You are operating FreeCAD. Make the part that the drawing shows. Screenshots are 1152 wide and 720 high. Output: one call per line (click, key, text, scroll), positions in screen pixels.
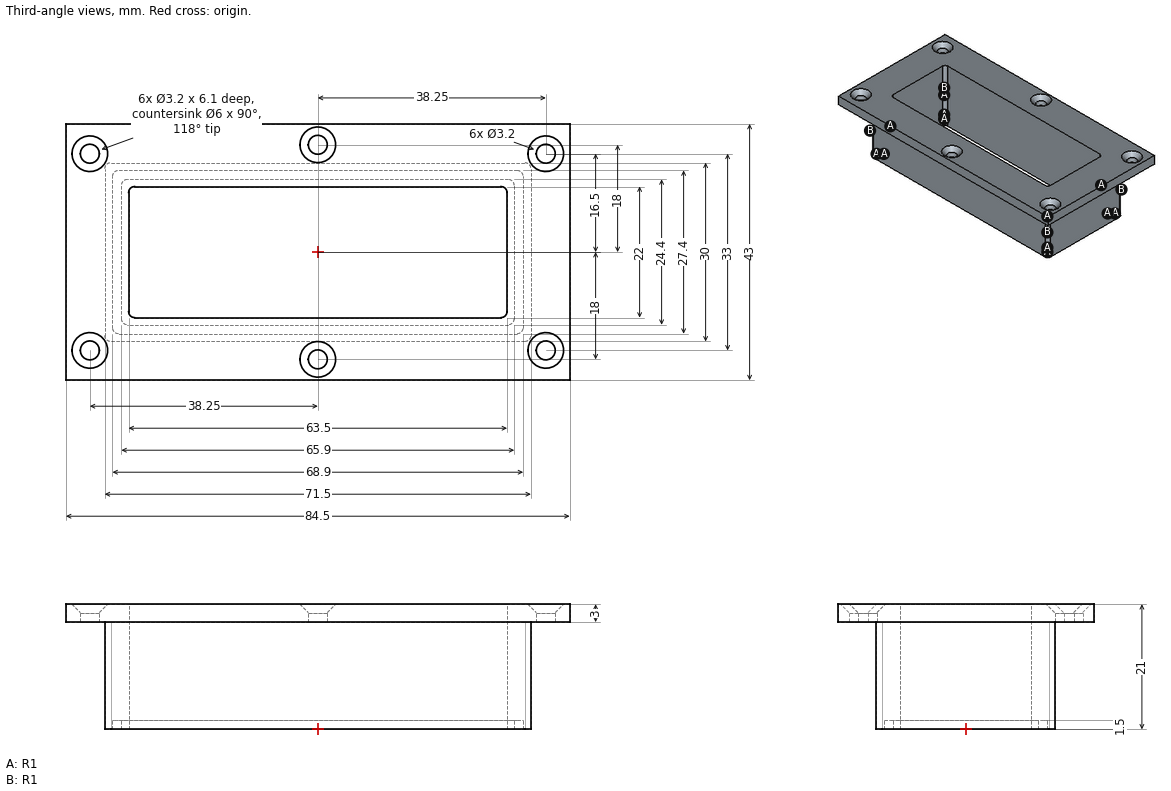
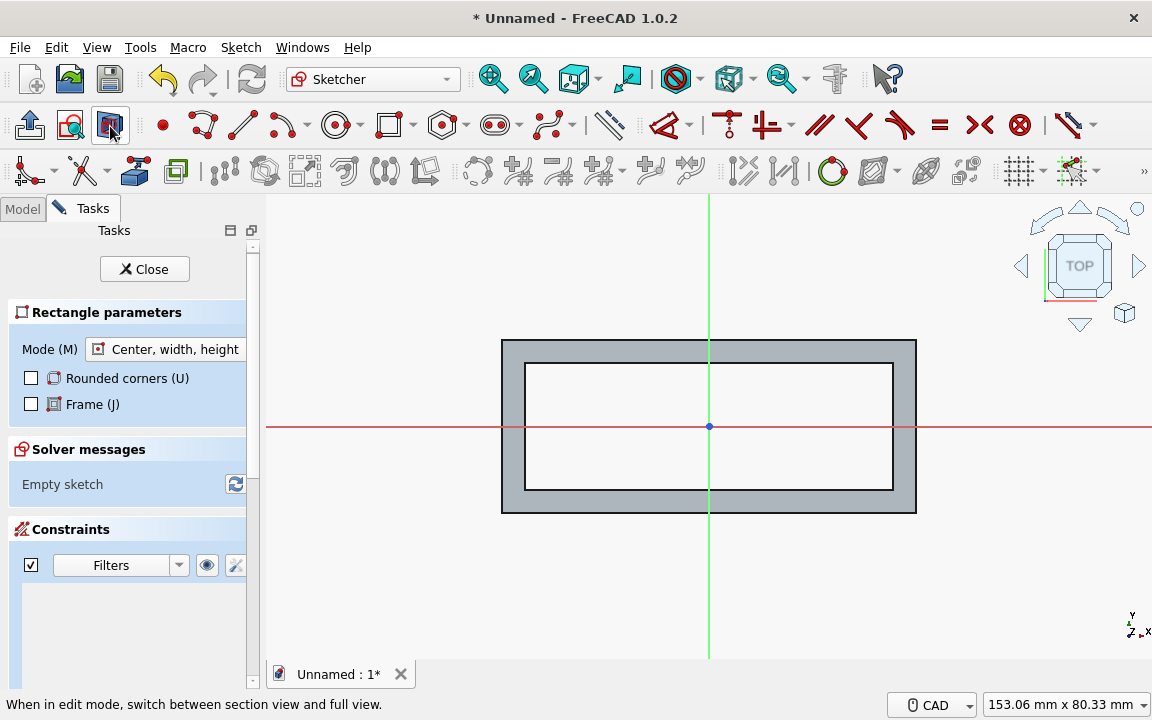
click(709, 426)
click(908, 347)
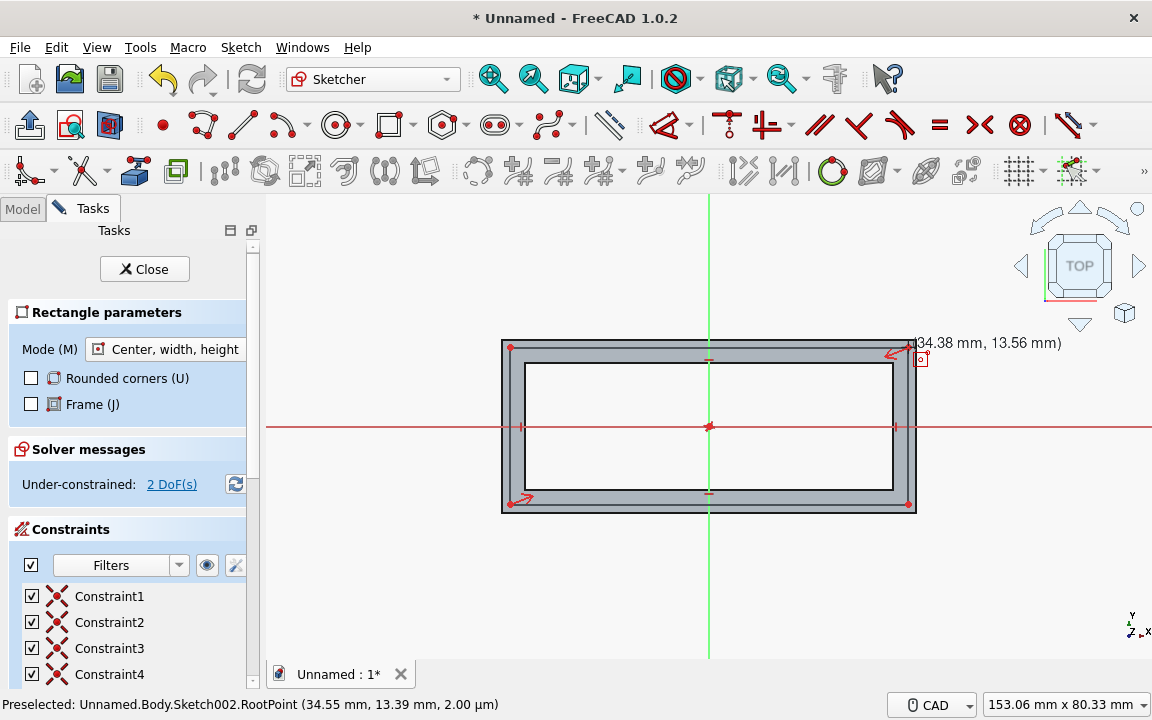
click(709, 426)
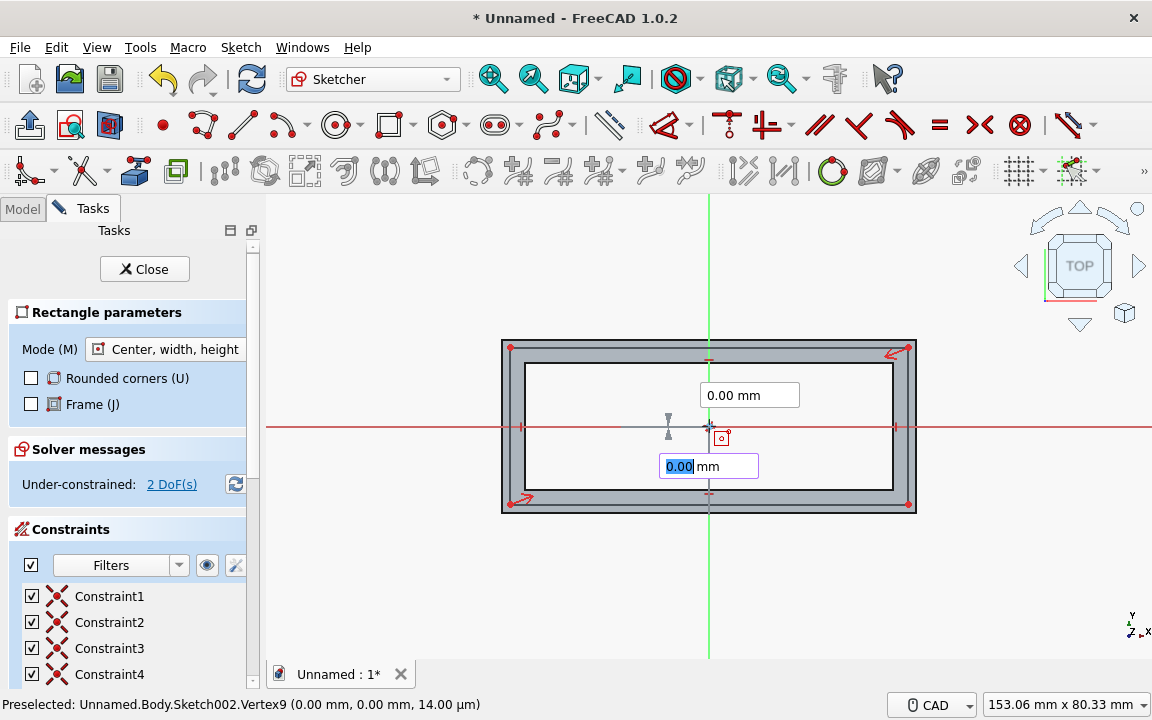
scroll(900, 356, up, 4)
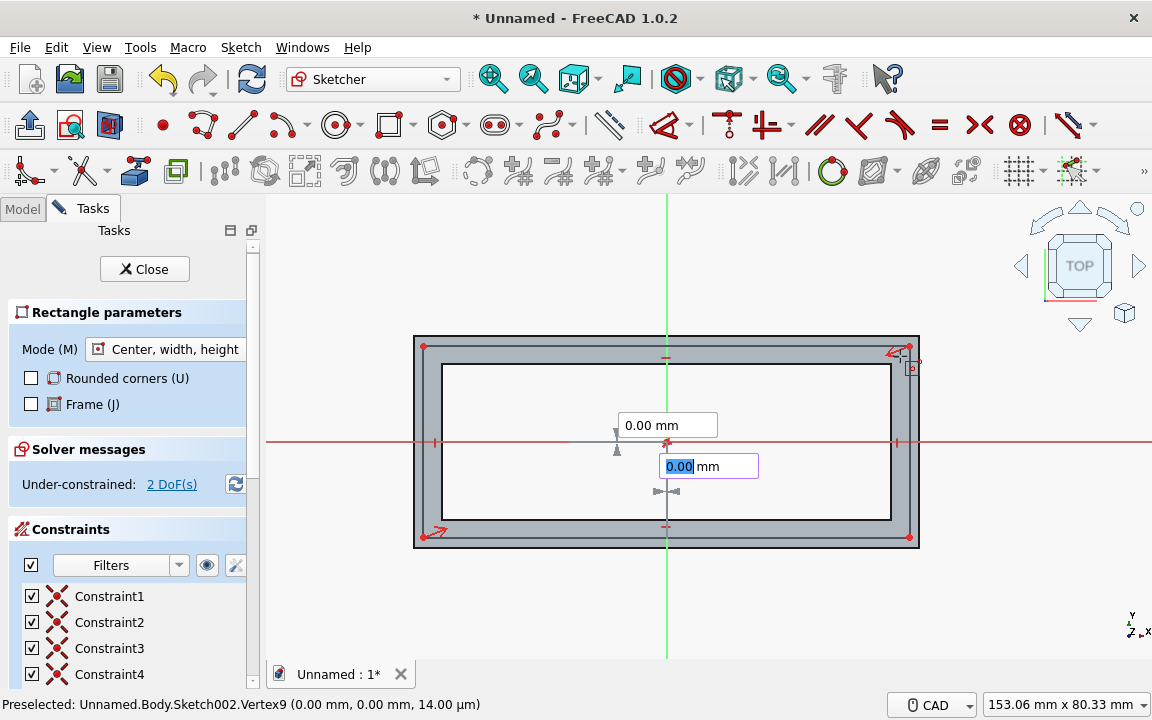
click(899, 355)
key(Escape)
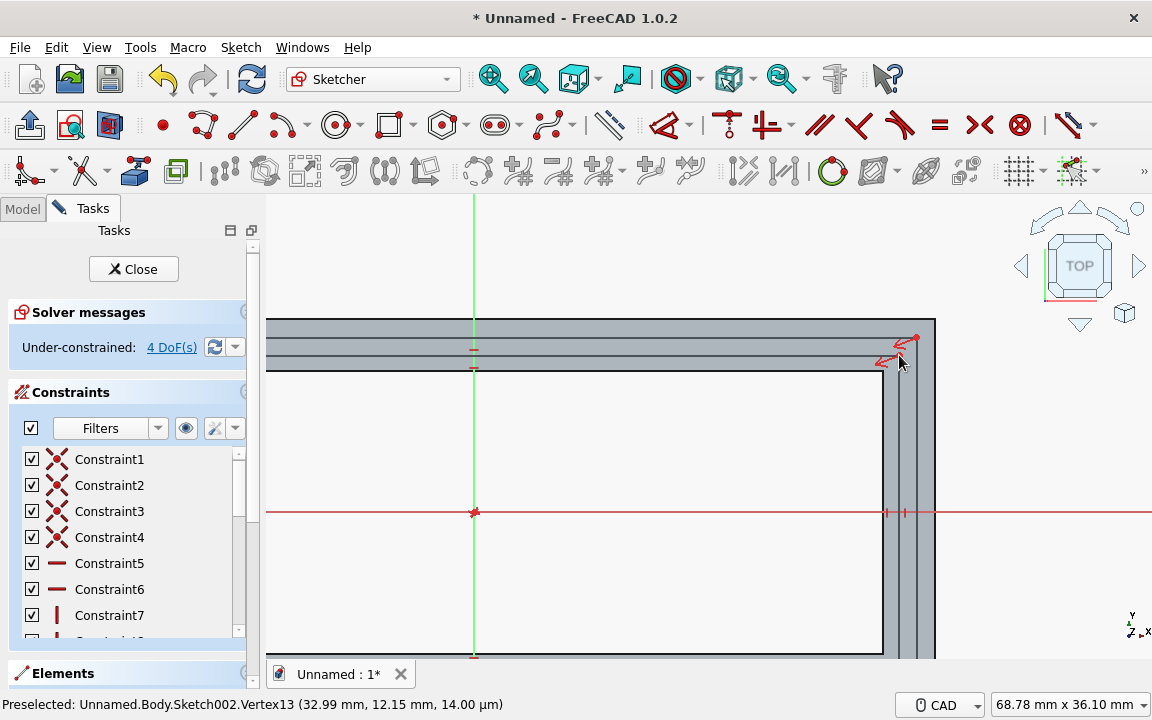
click(664, 126)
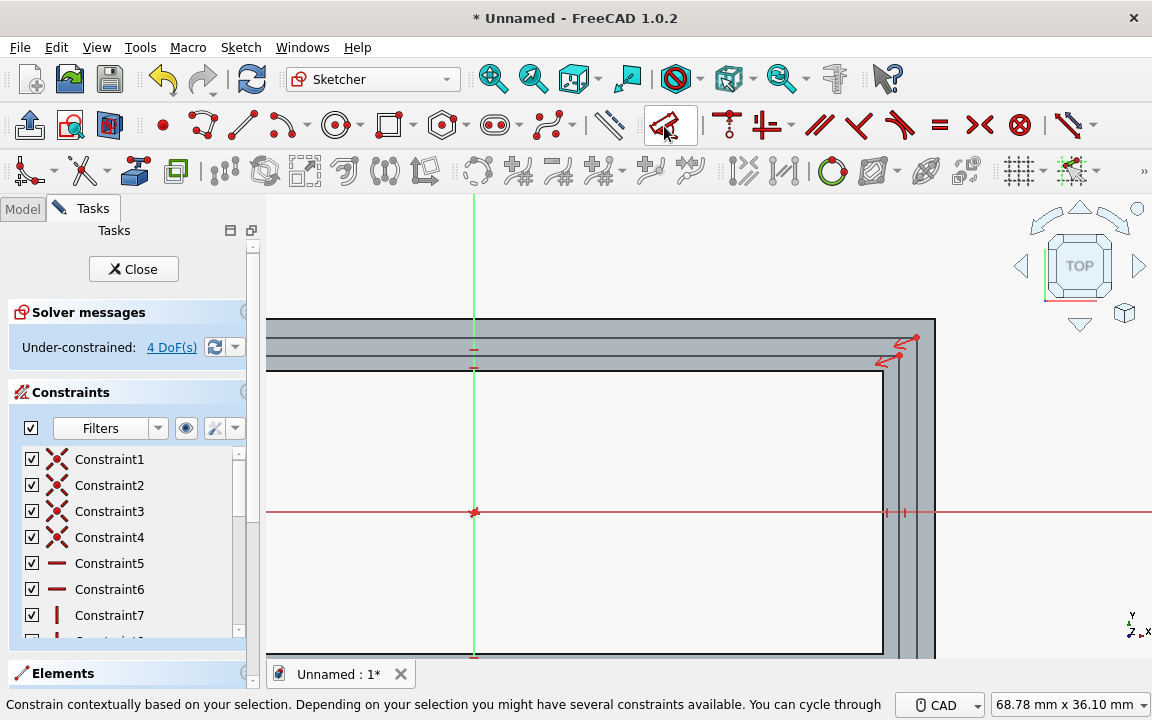
scroll(843, 322, down, 3)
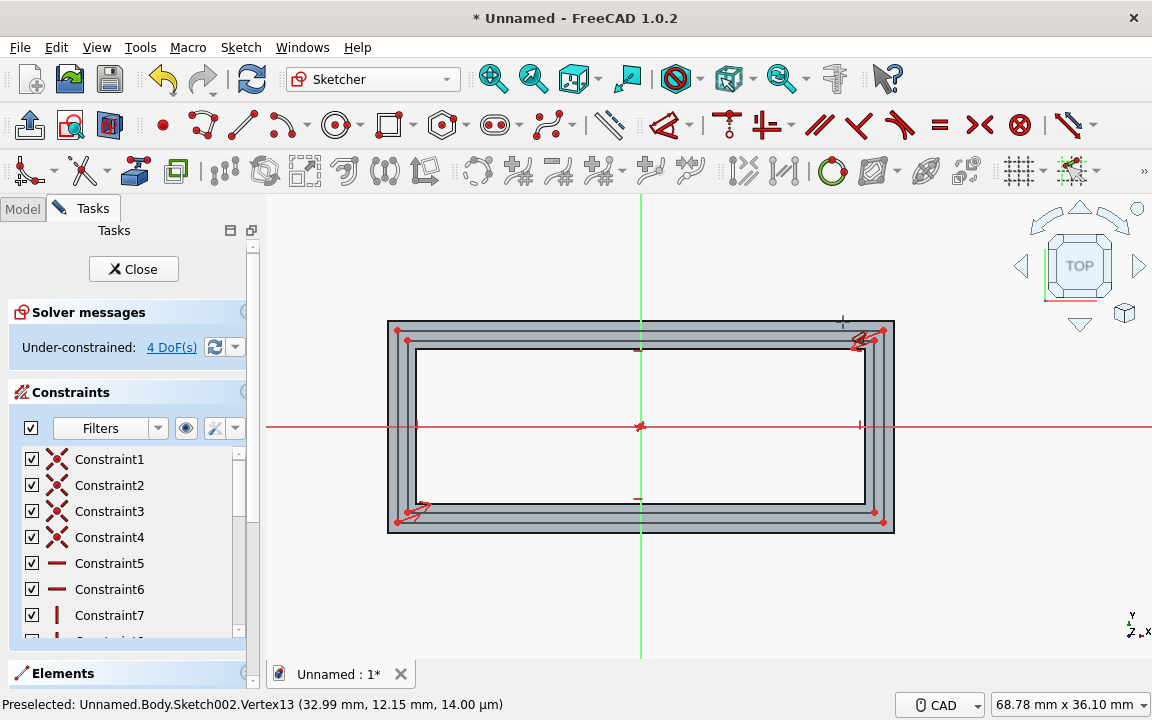
scroll(544, 523, up, 2)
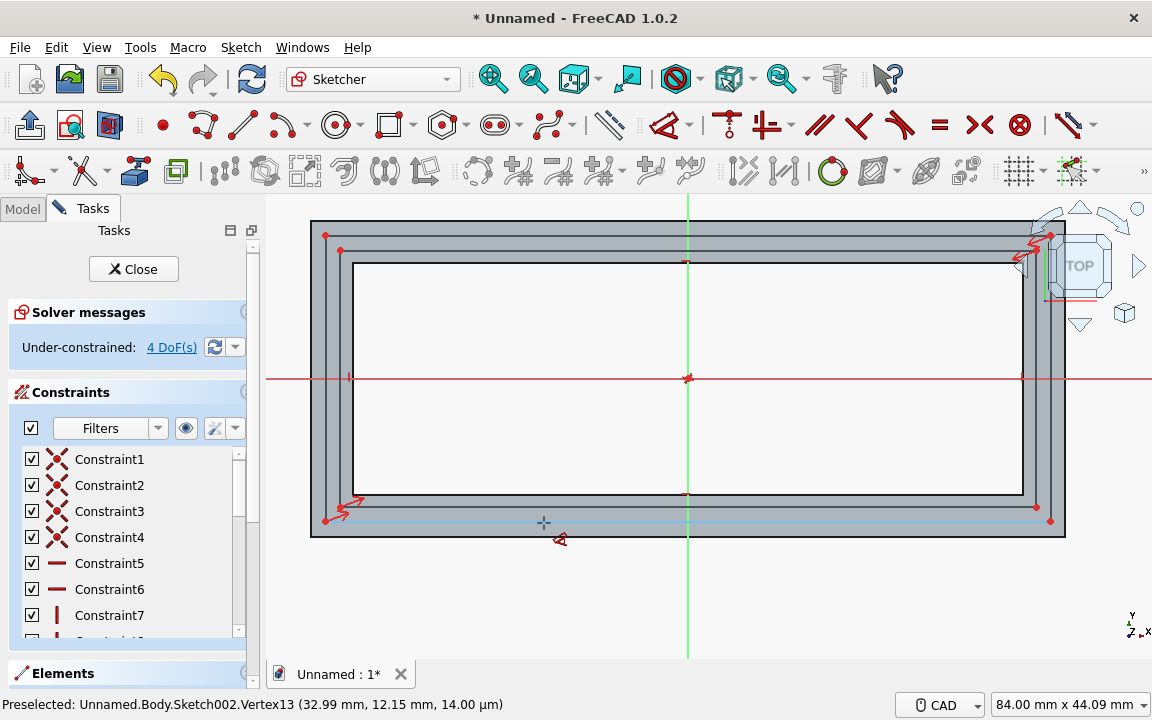
click(543, 522)
click(656, 556)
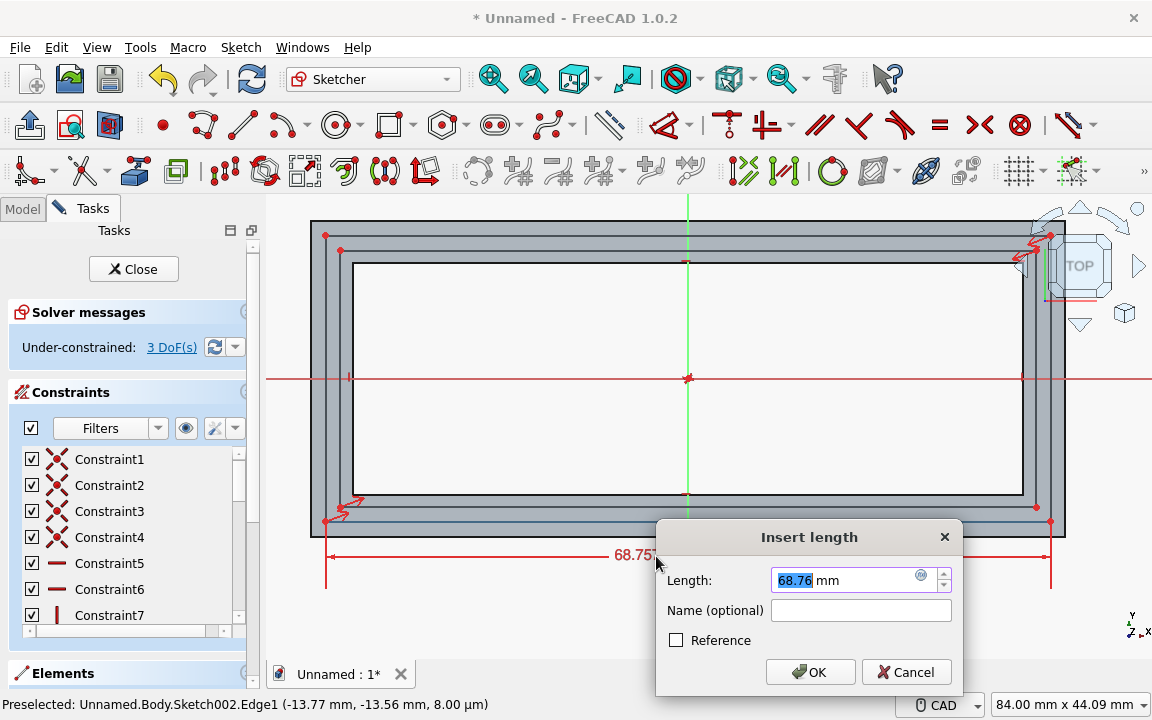
text(68.9)
key(Return)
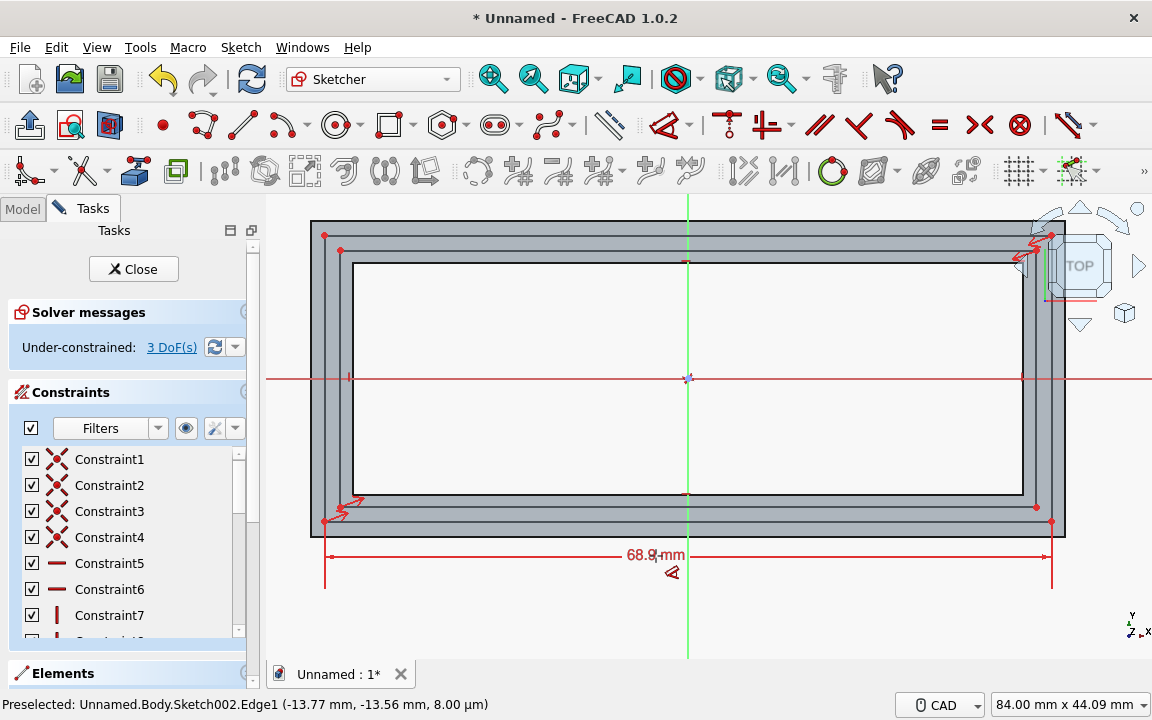
scroll(543, 523, down, 2)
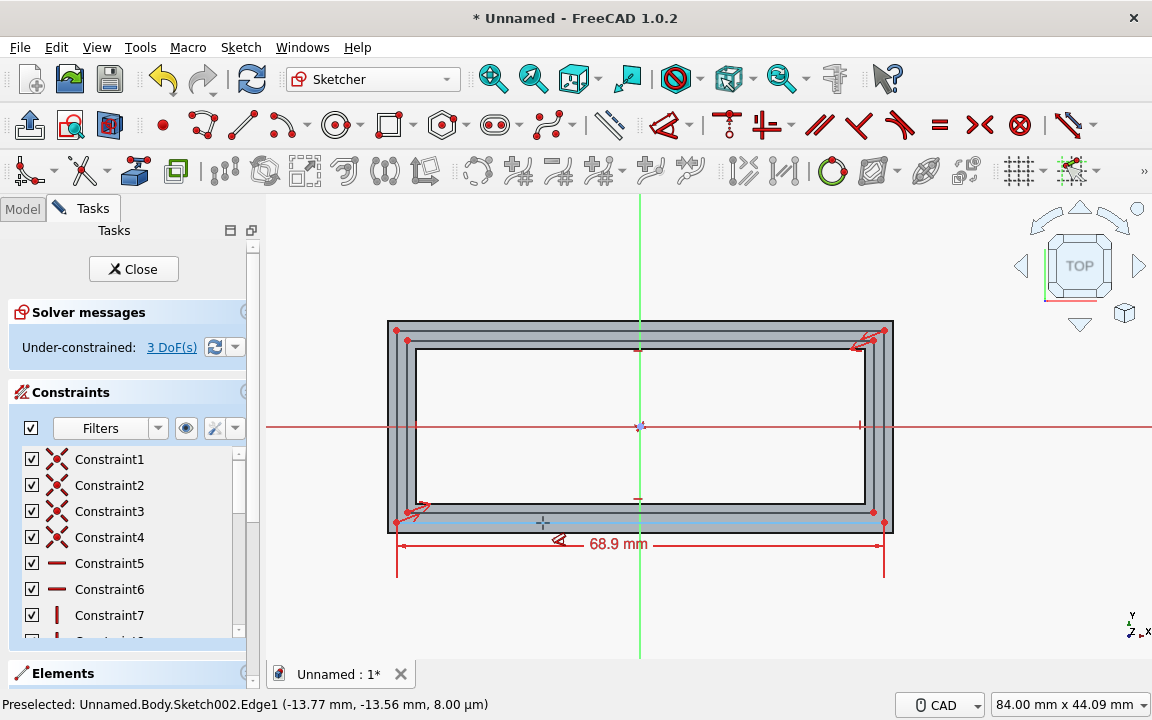
scroll(884, 465, up, 2)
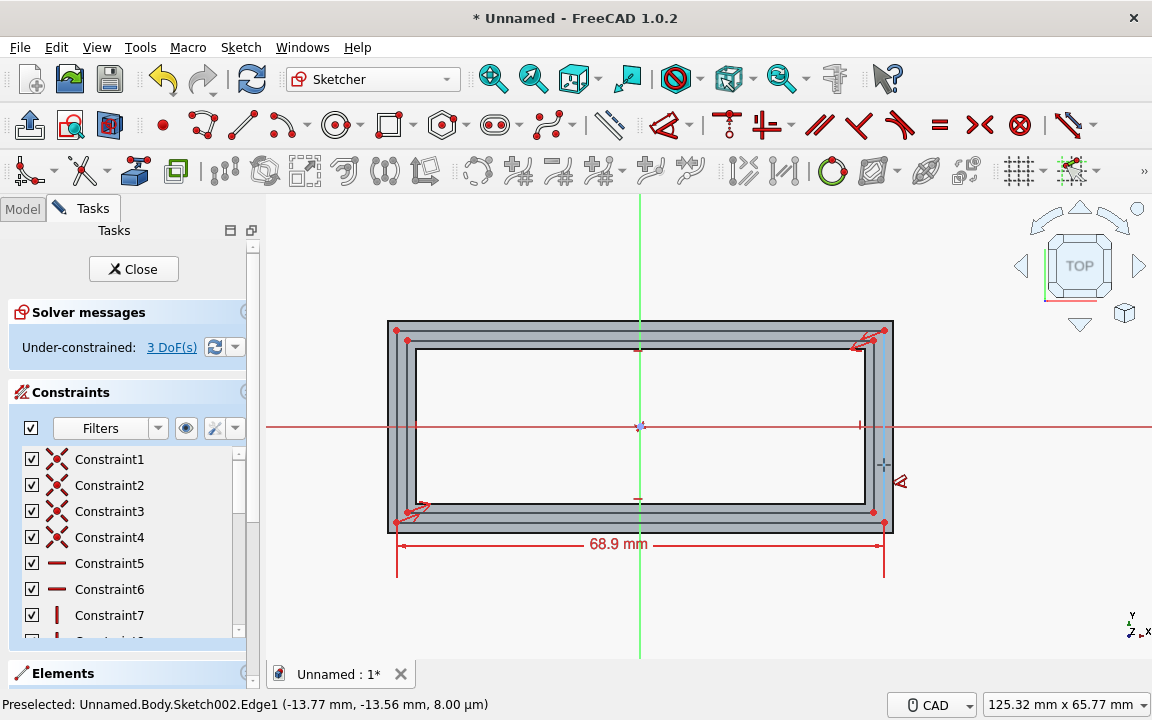
click(884, 465)
click(918, 342)